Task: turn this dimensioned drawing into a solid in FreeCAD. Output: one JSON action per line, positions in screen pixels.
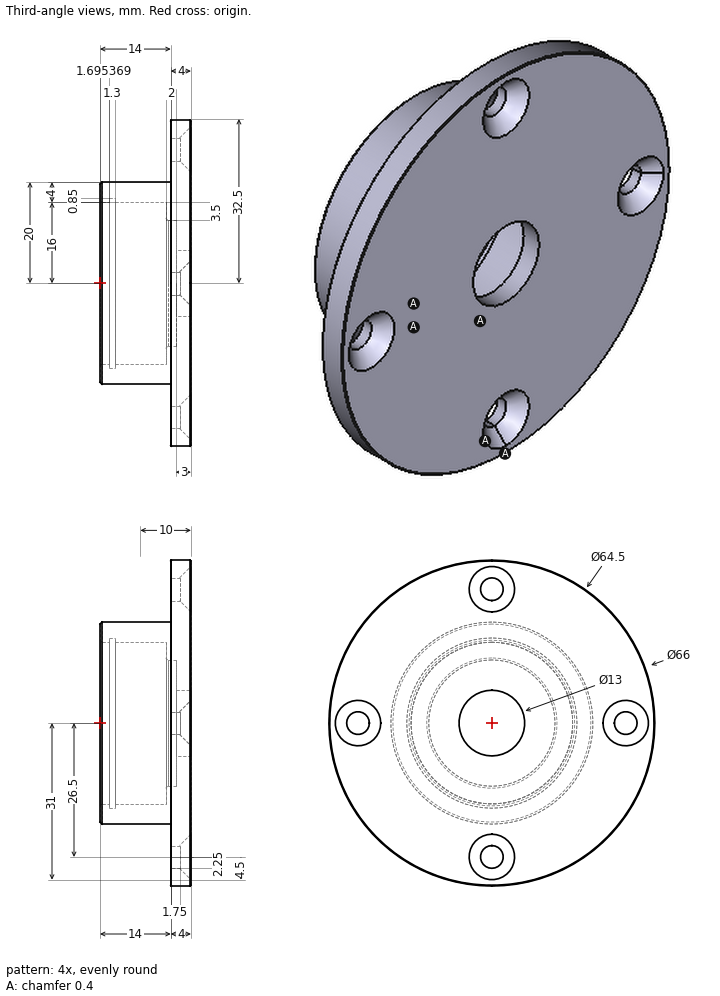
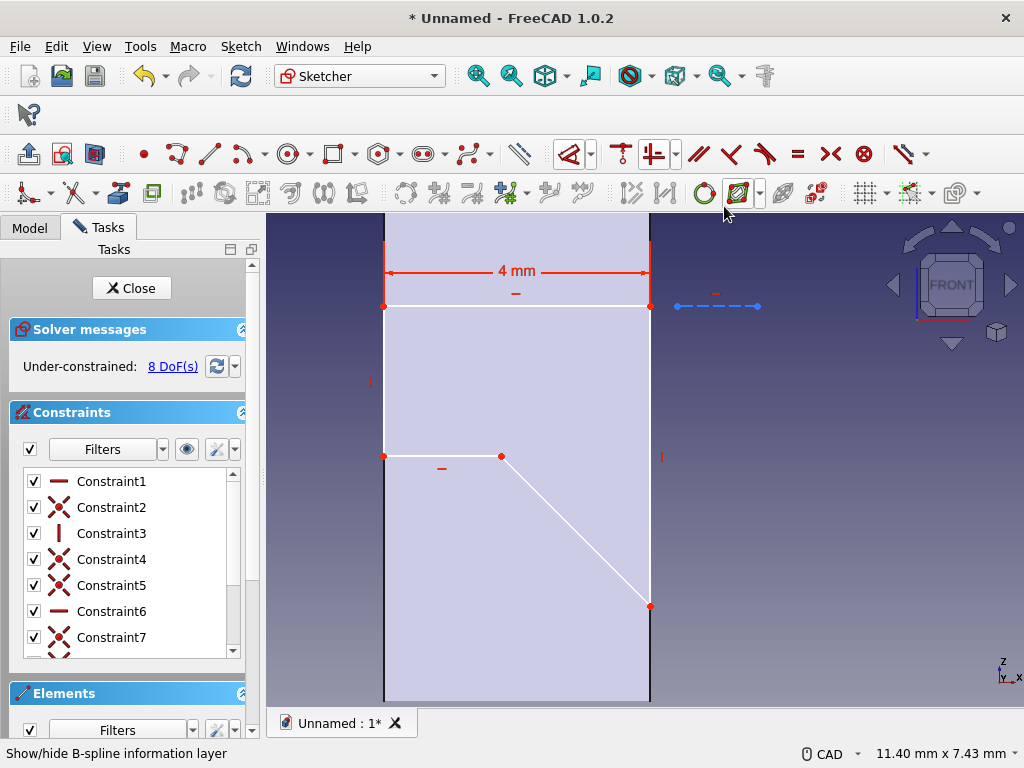
{"action": "left_click", "coordinate": [650, 396]}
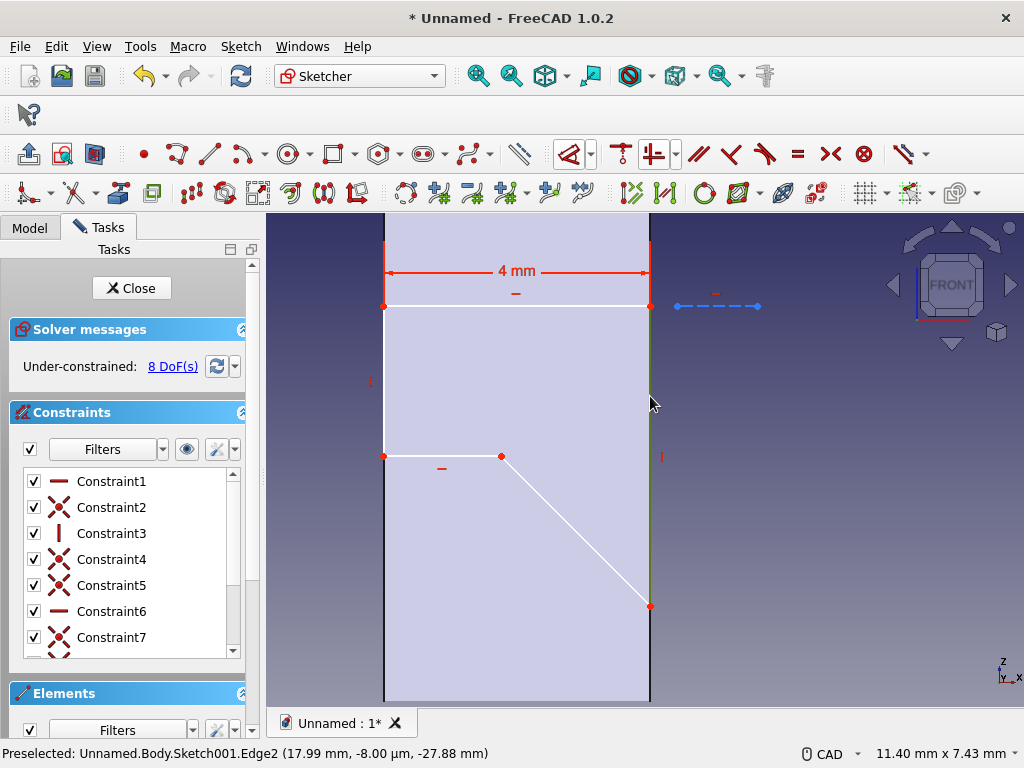
{"action": "key", "text": "i"}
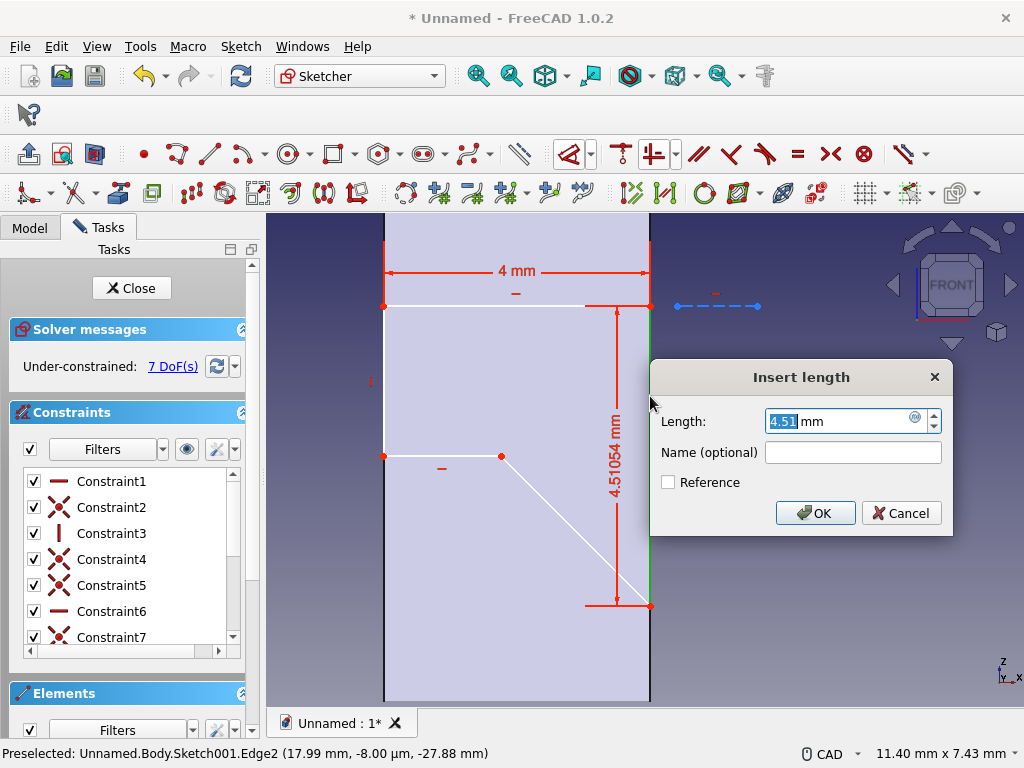
{"action": "type", "text": "4.5"}
{"action": "key", "text": "Return"}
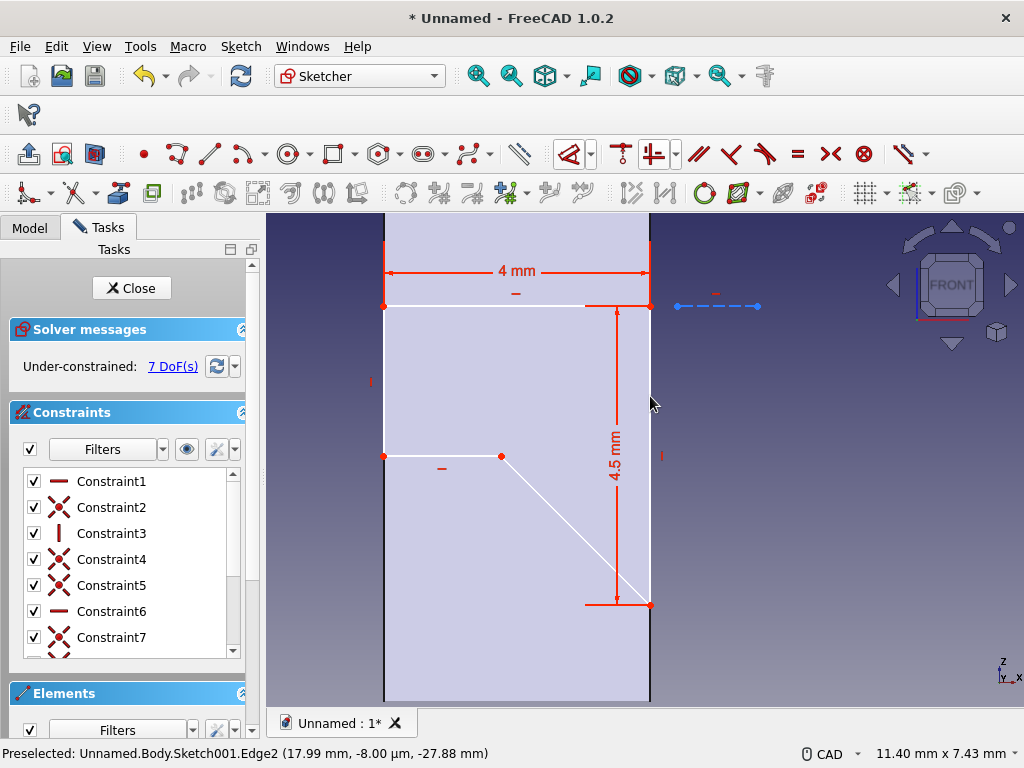
{"action": "left_click", "coordinate": [384, 306]}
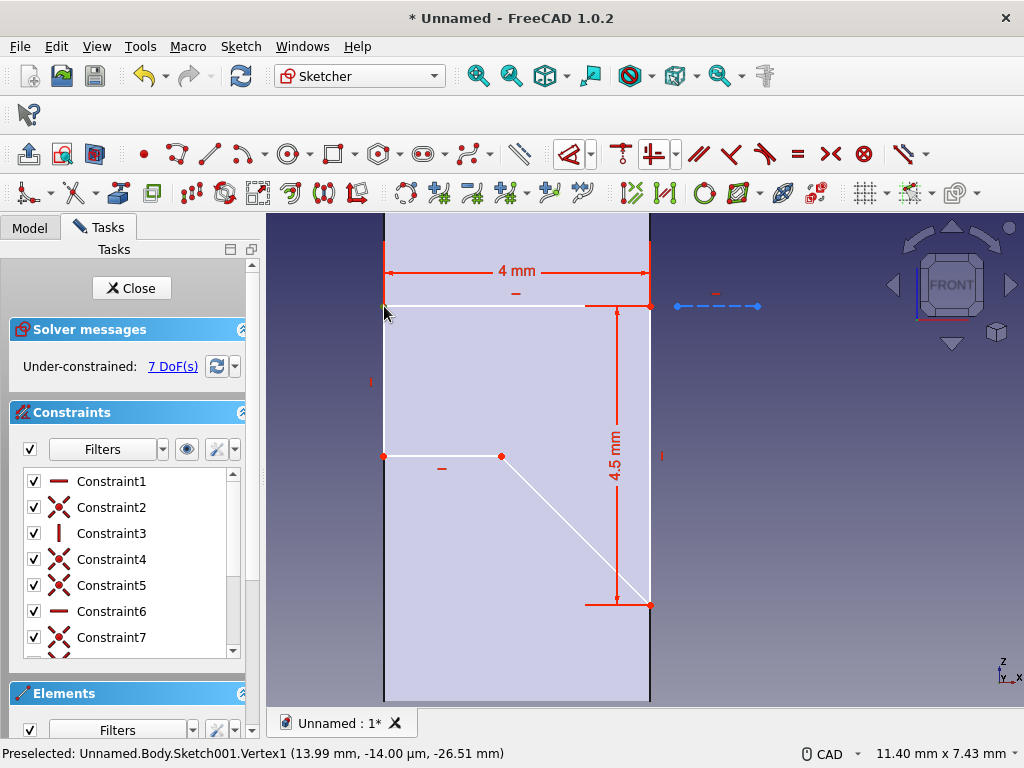
{"action": "left_click", "coordinate": [590, 154]}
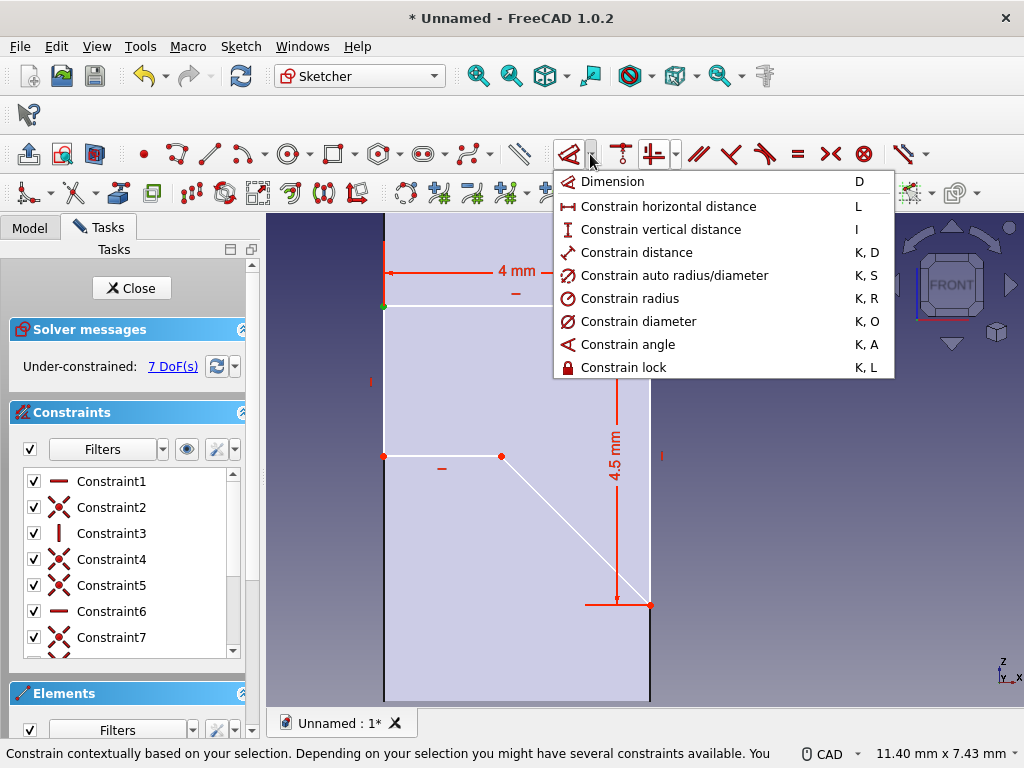
{"action": "left_click", "coordinate": [724, 206]}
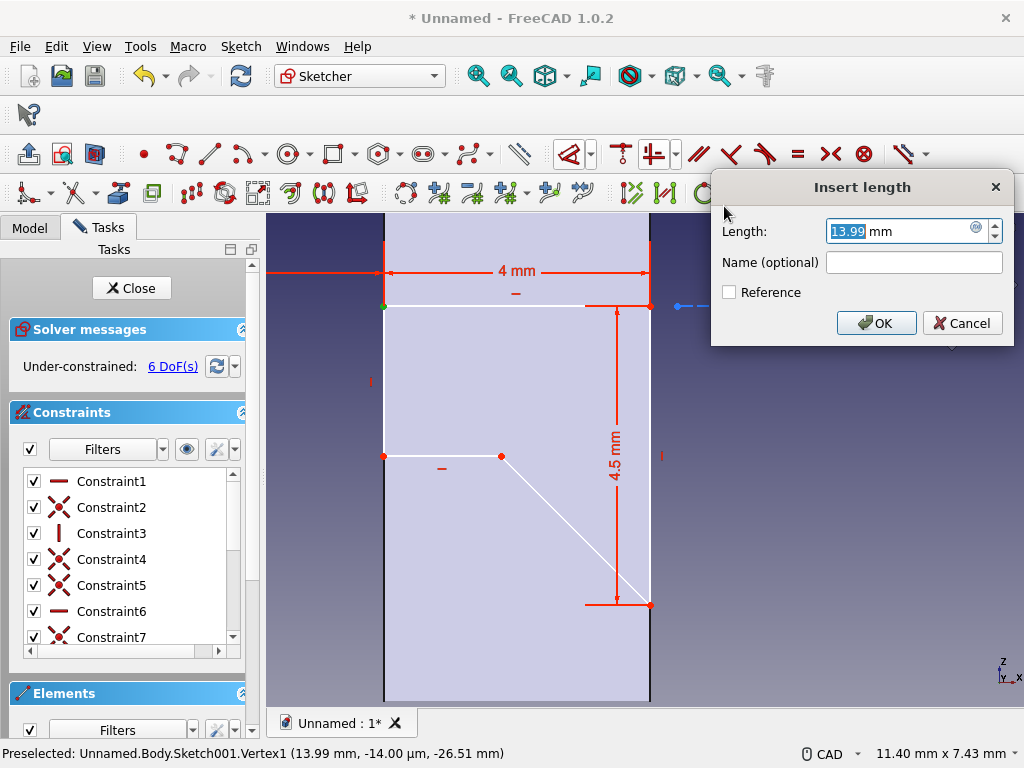
{"action": "type", "text": "14"}
{"action": "key", "text": "Return"}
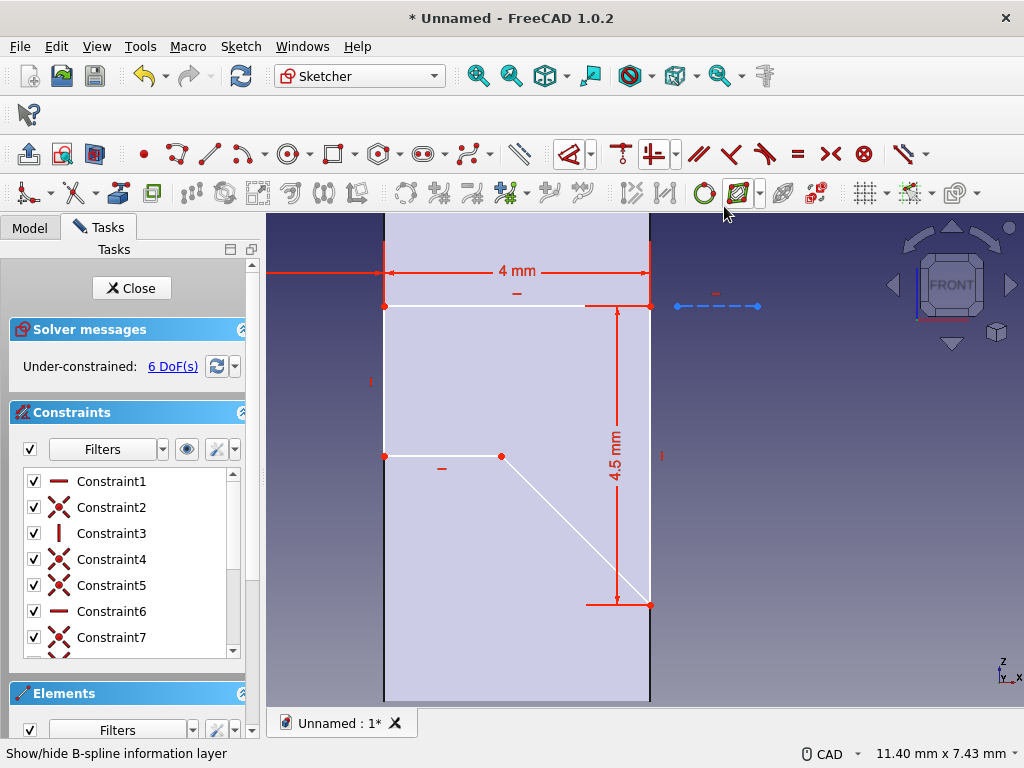
{"action": "left_click", "coordinate": [650, 605]}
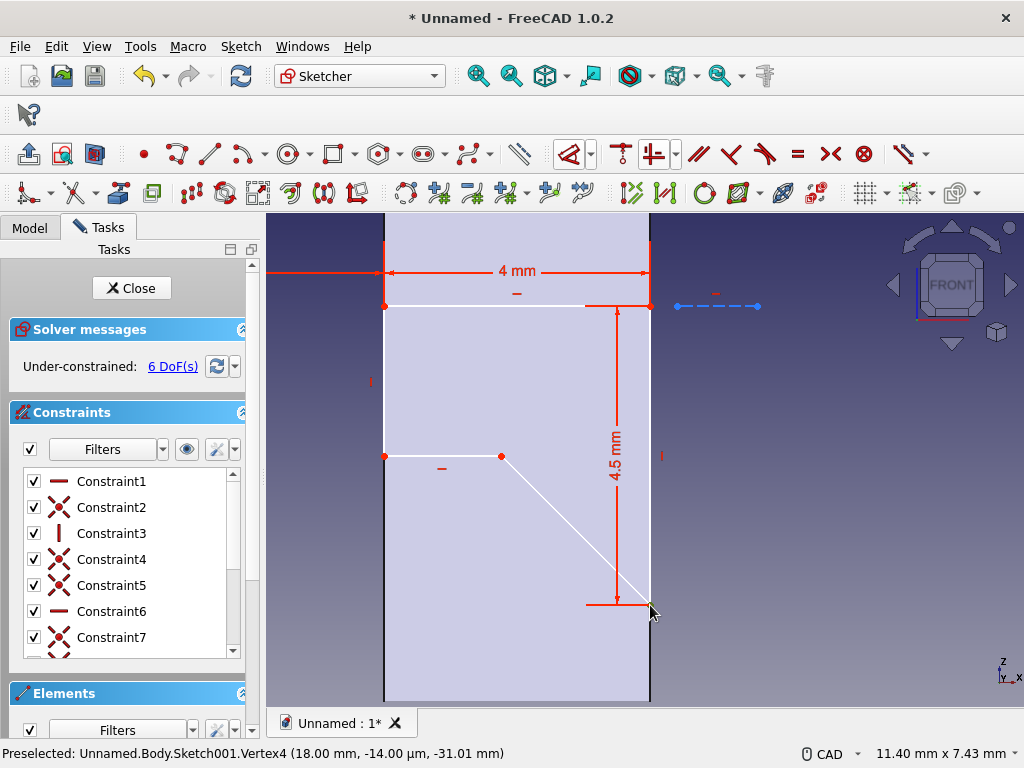
{"action": "left_click", "coordinate": [590, 154]}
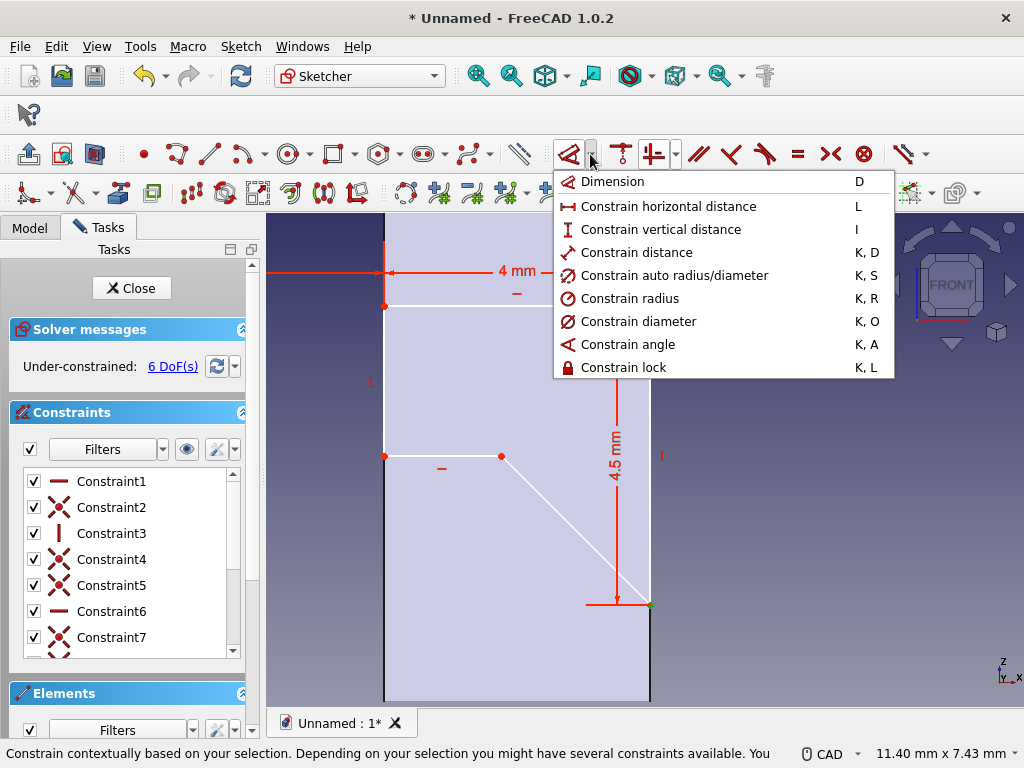
{"action": "left_click", "coordinate": [724, 230]}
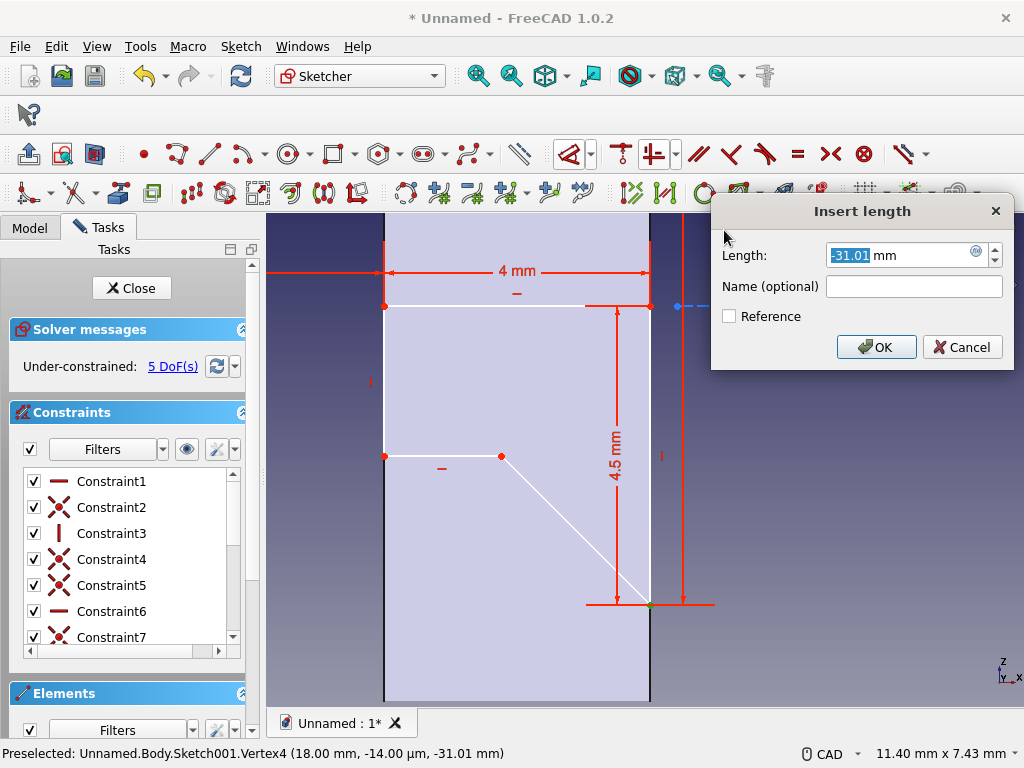
{"action": "type", "text": "-31"}
{"action": "key", "text": "Return"}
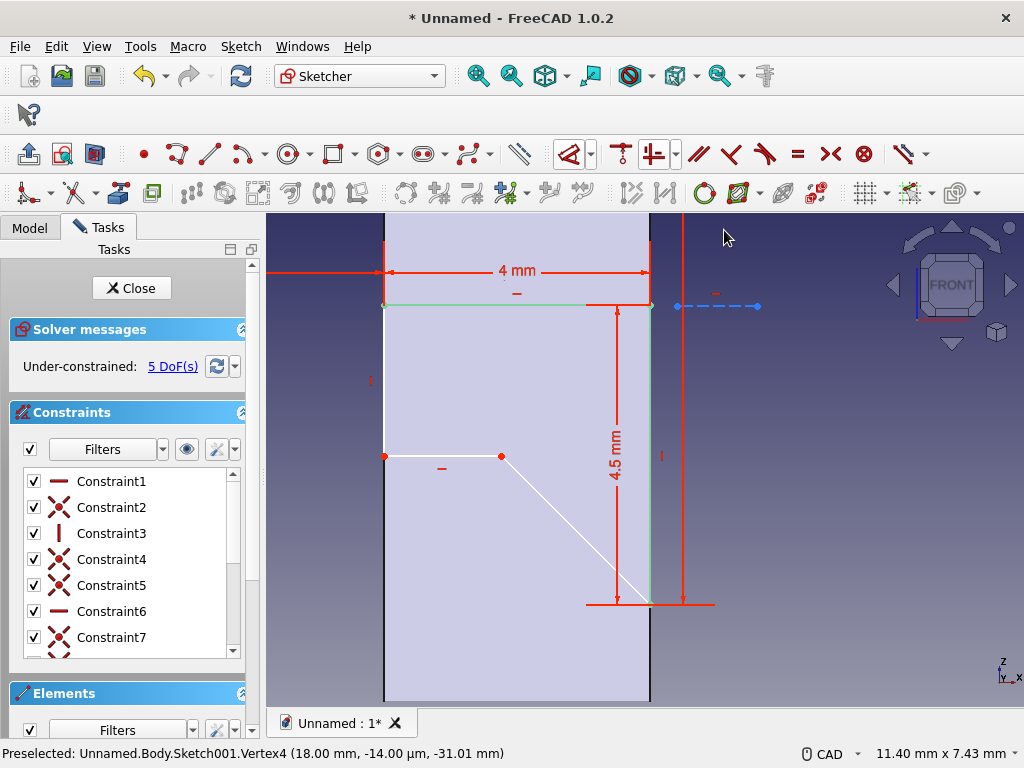
{"action": "left_click", "coordinate": [466, 456]}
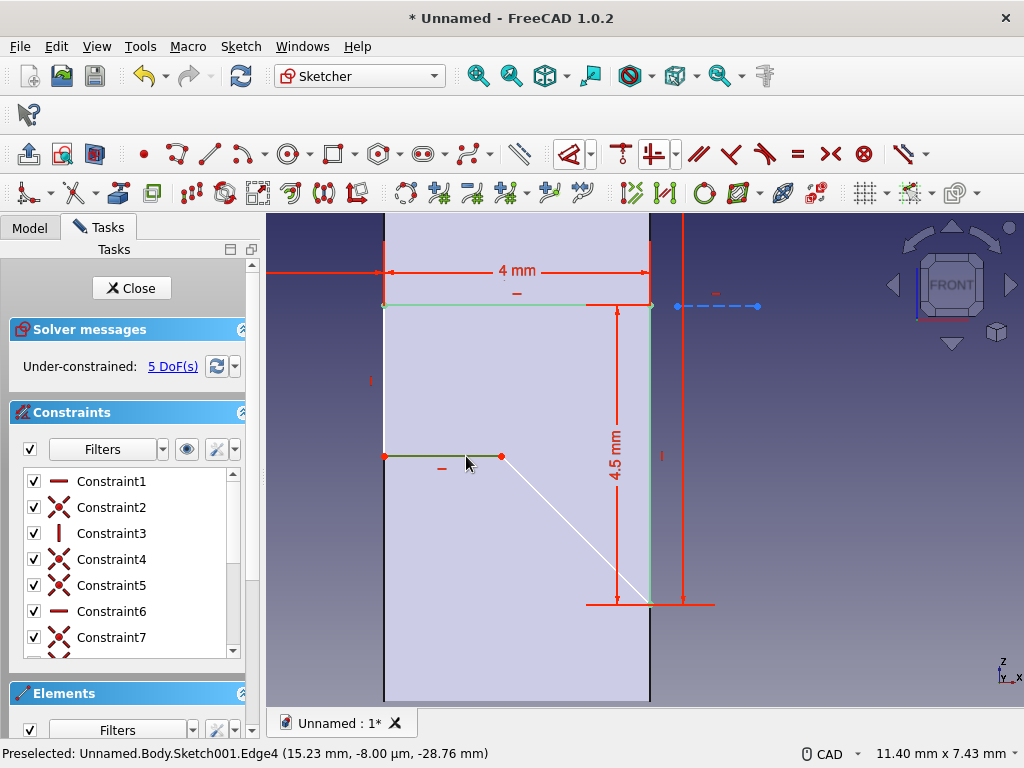
{"action": "left_click", "coordinate": [590, 154]}